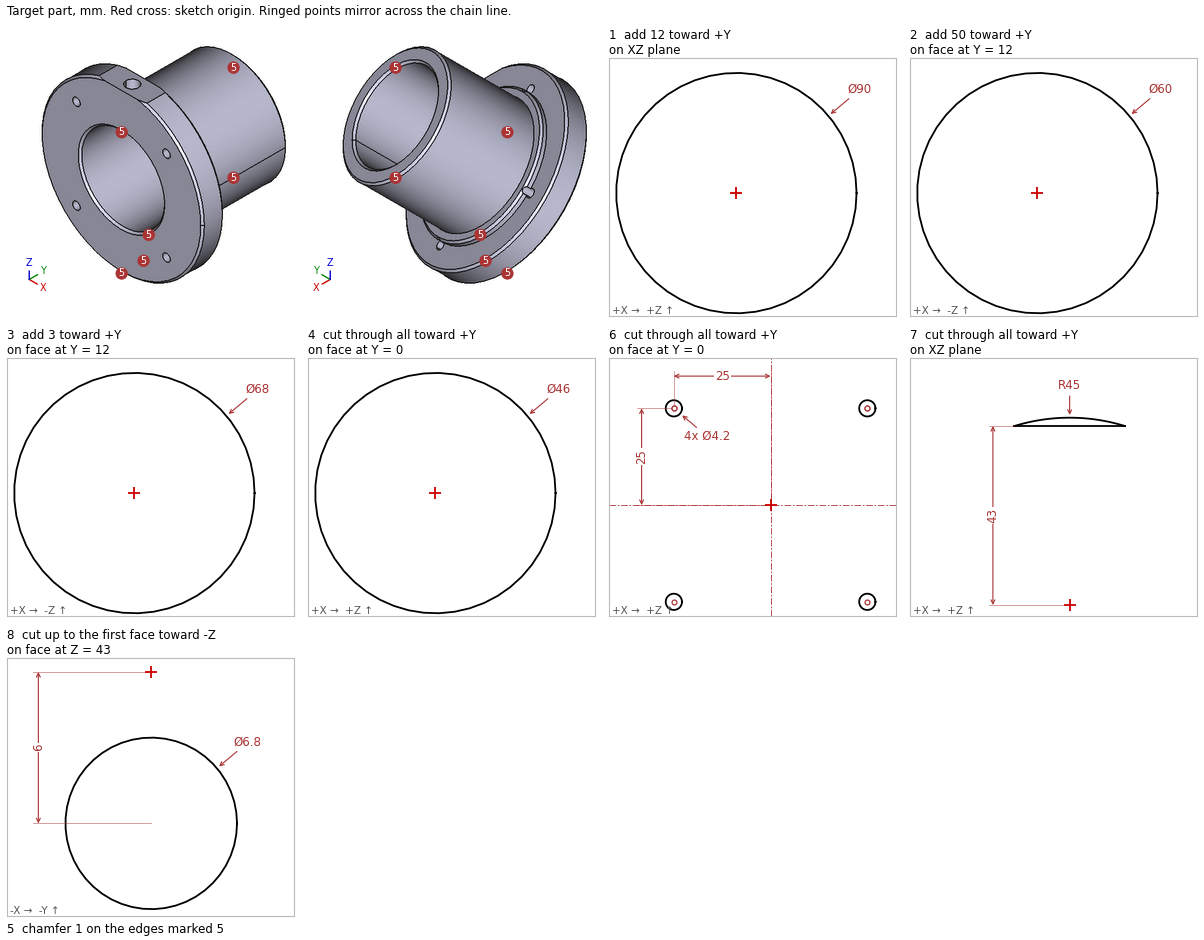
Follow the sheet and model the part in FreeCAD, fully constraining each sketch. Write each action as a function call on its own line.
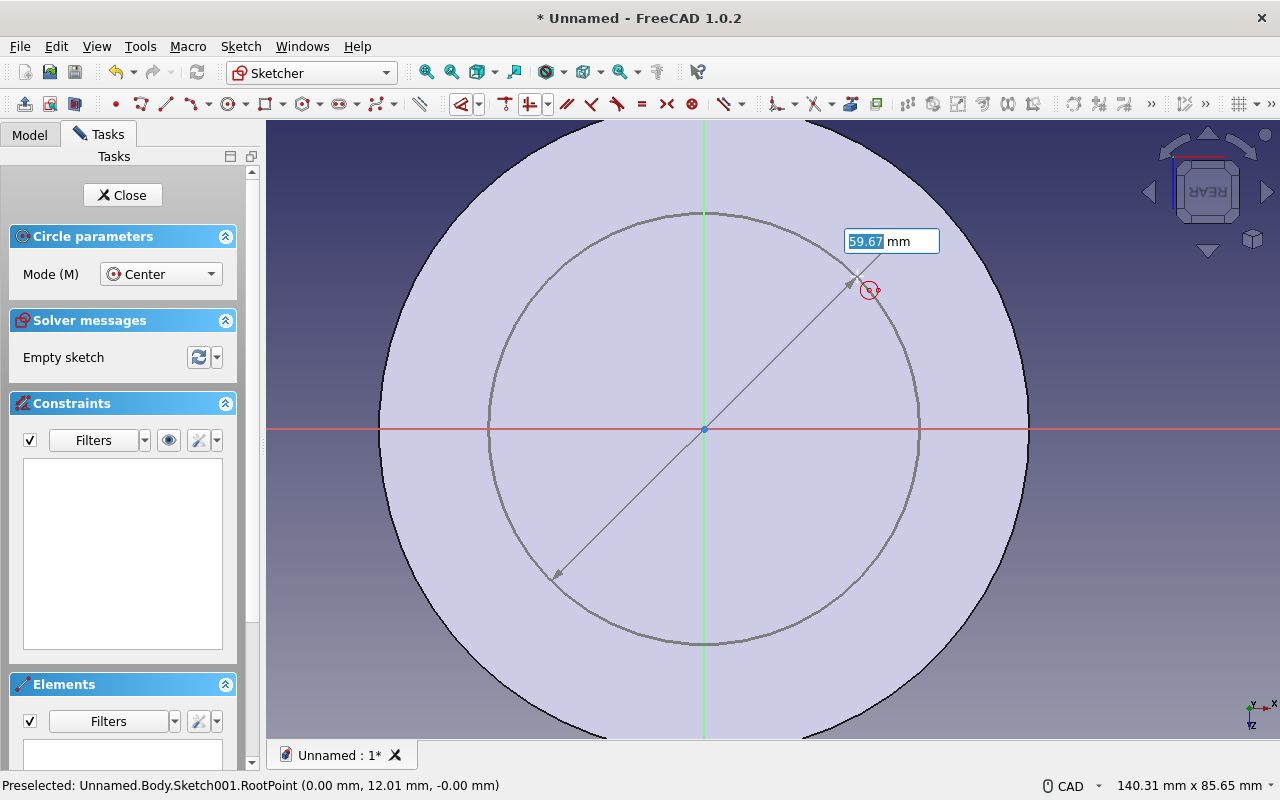
text(60)
key(Return)
key(Escape)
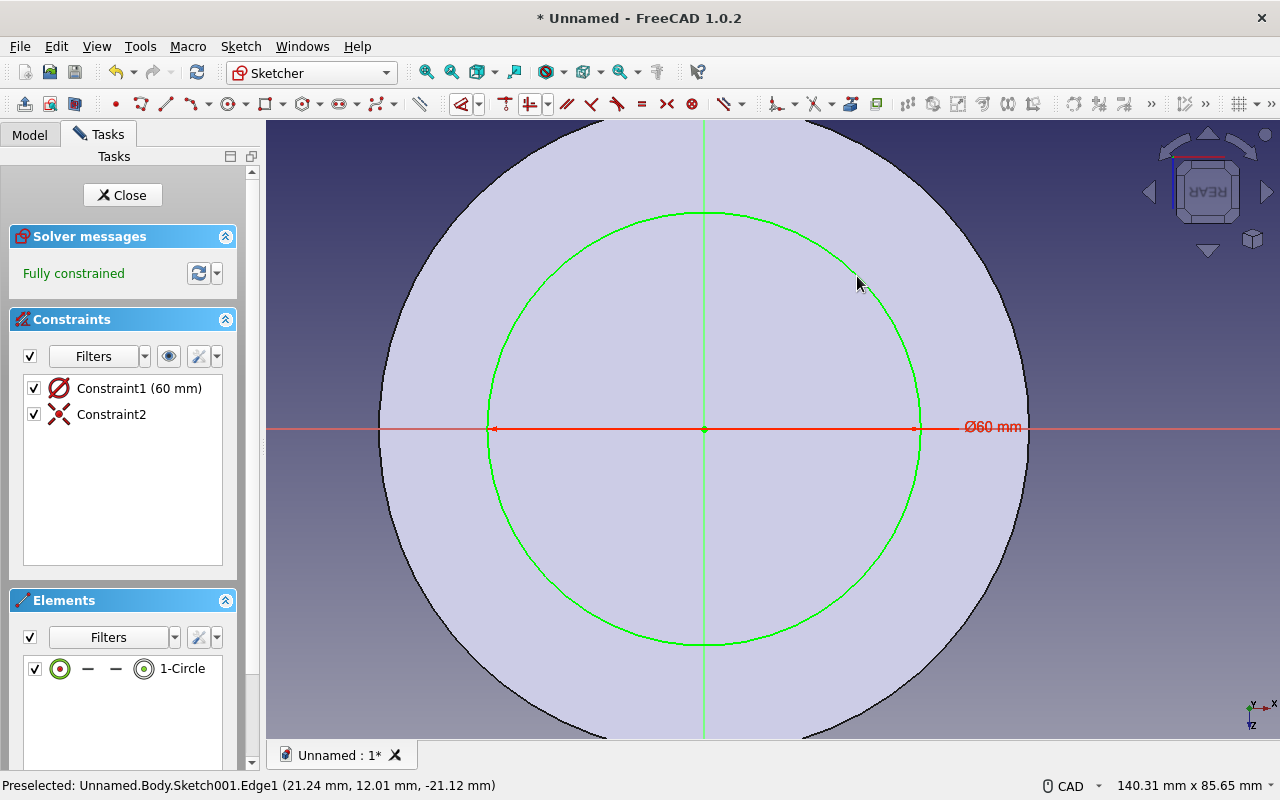
click(123, 195)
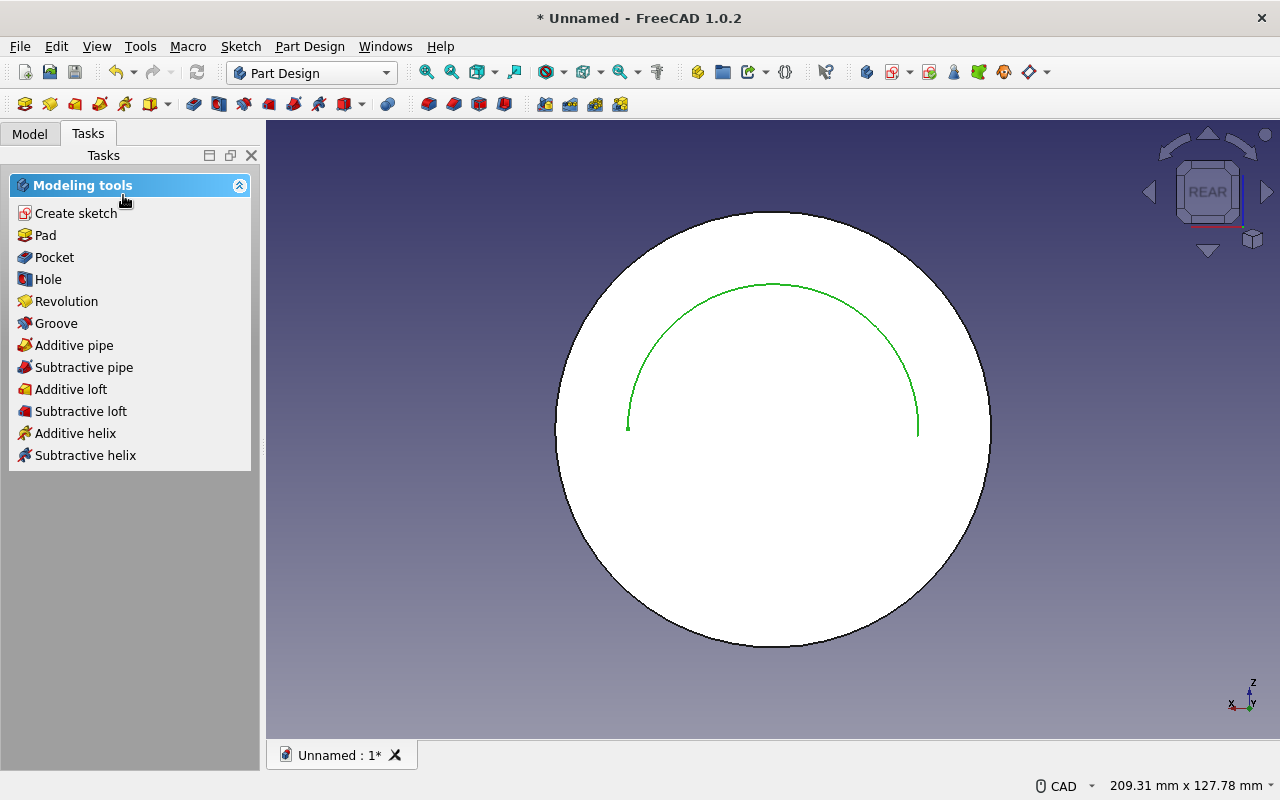
click(25, 104)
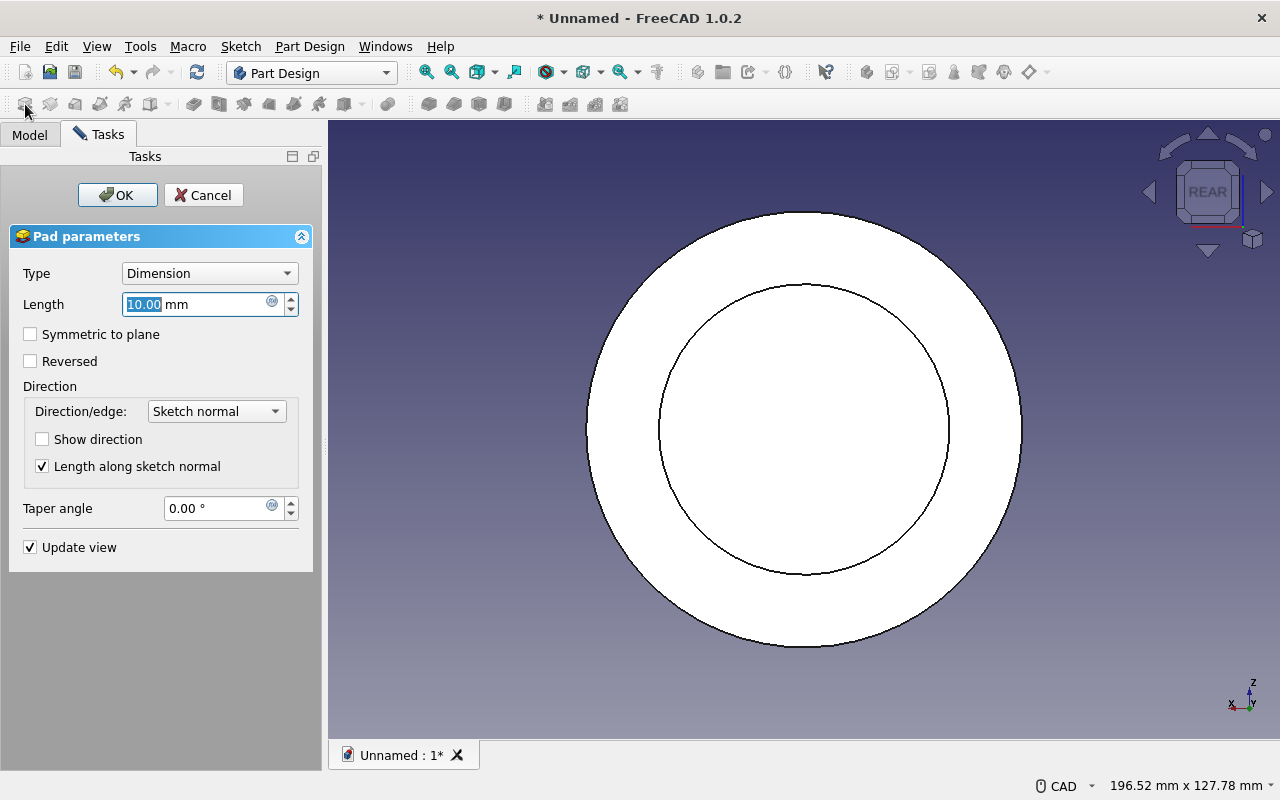
text(50)
key(Tab)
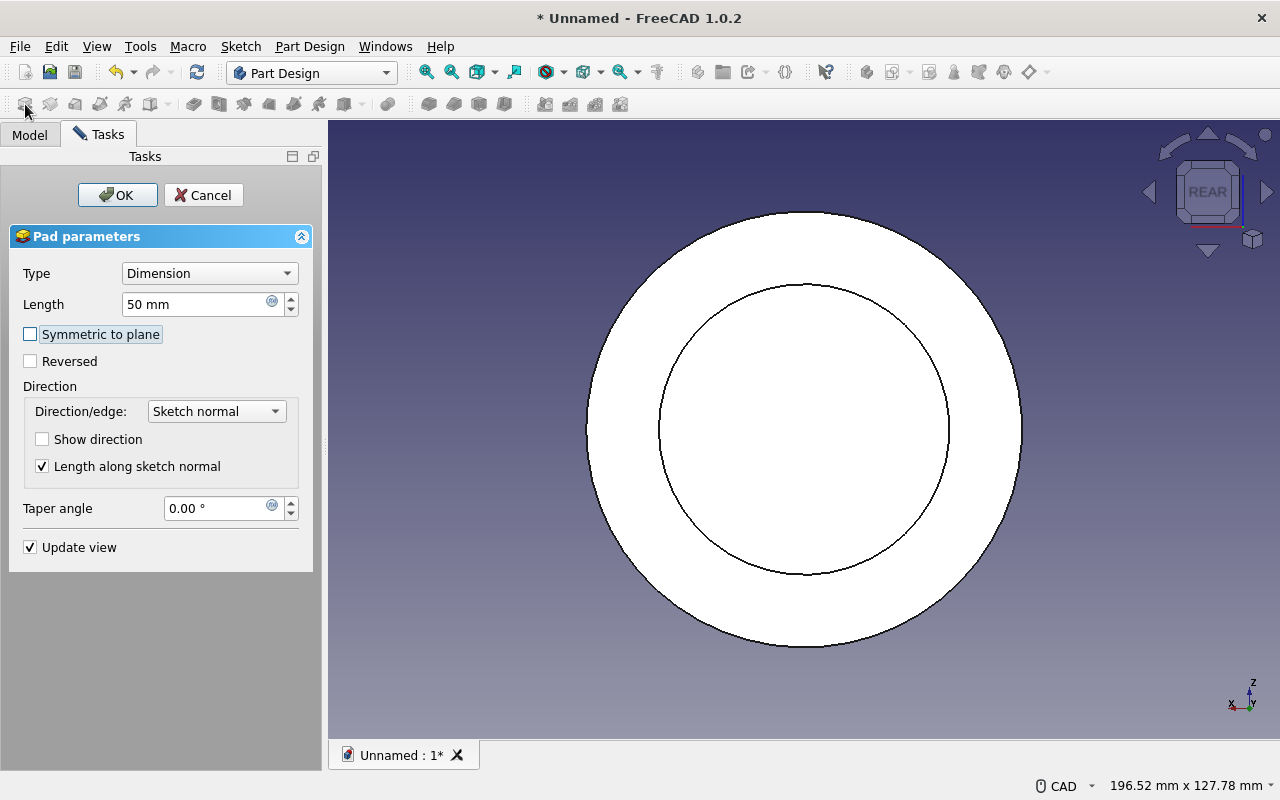
click(118, 195)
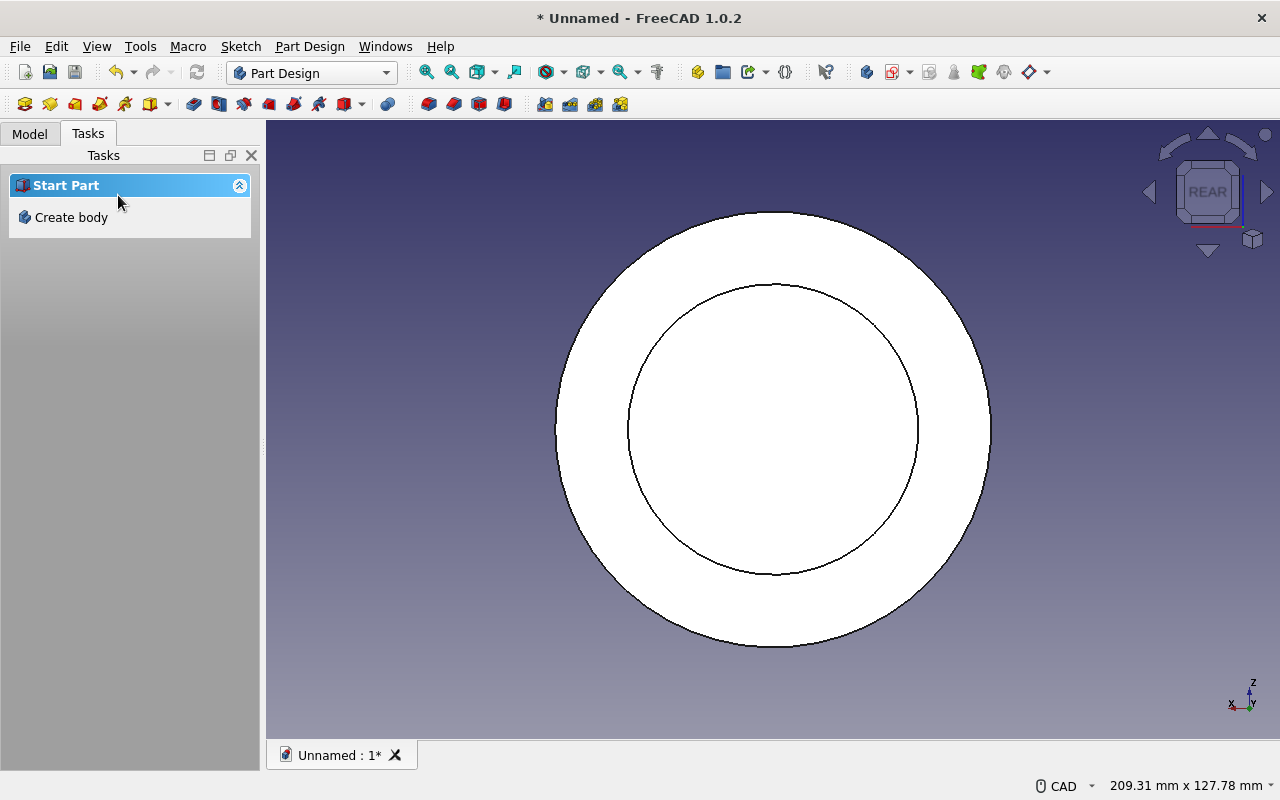
click(586, 428)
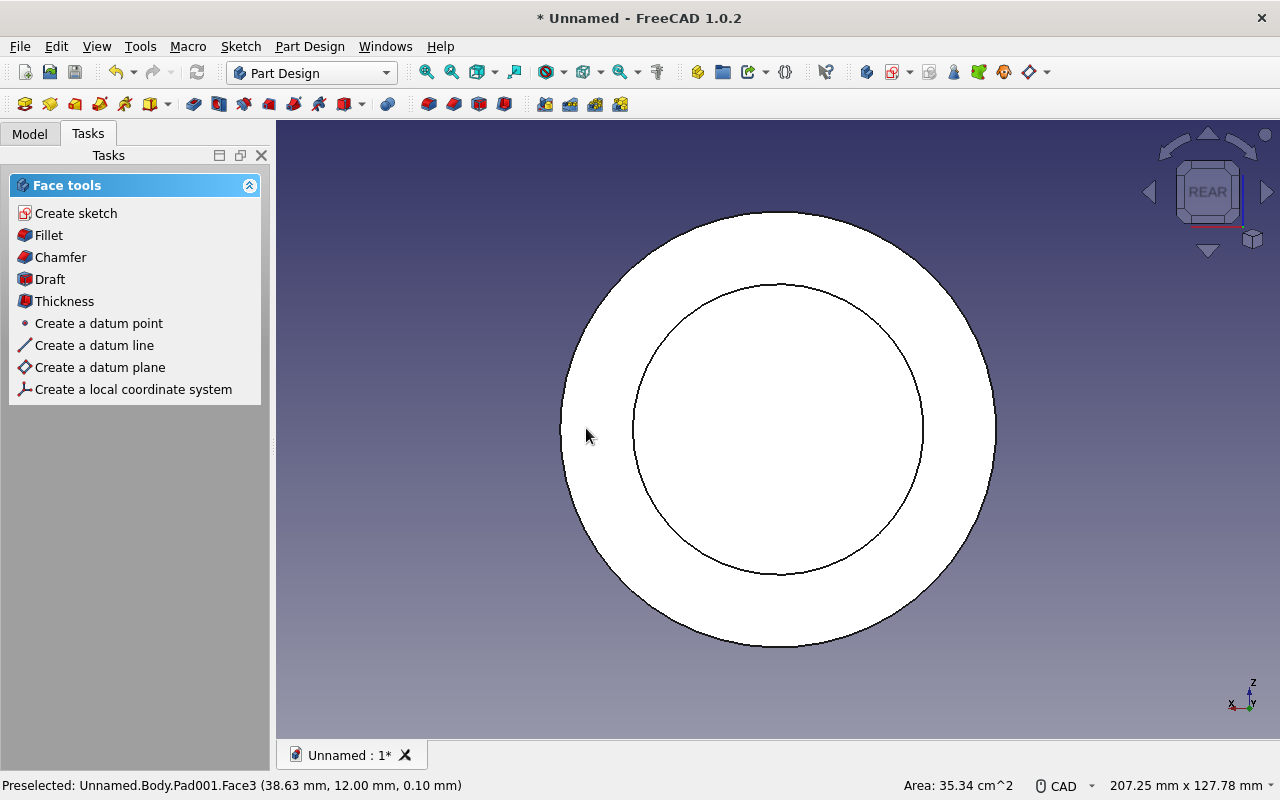
click(892, 72)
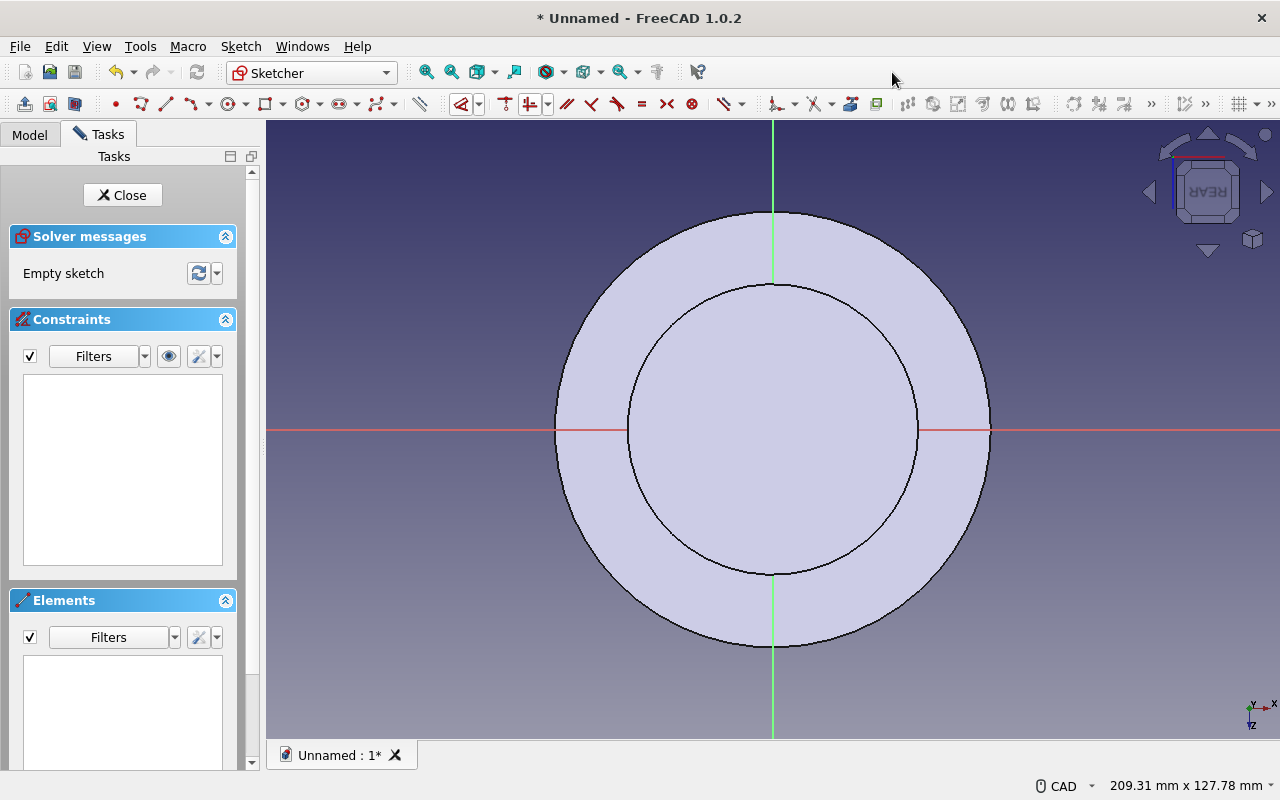
key(g)
key(c)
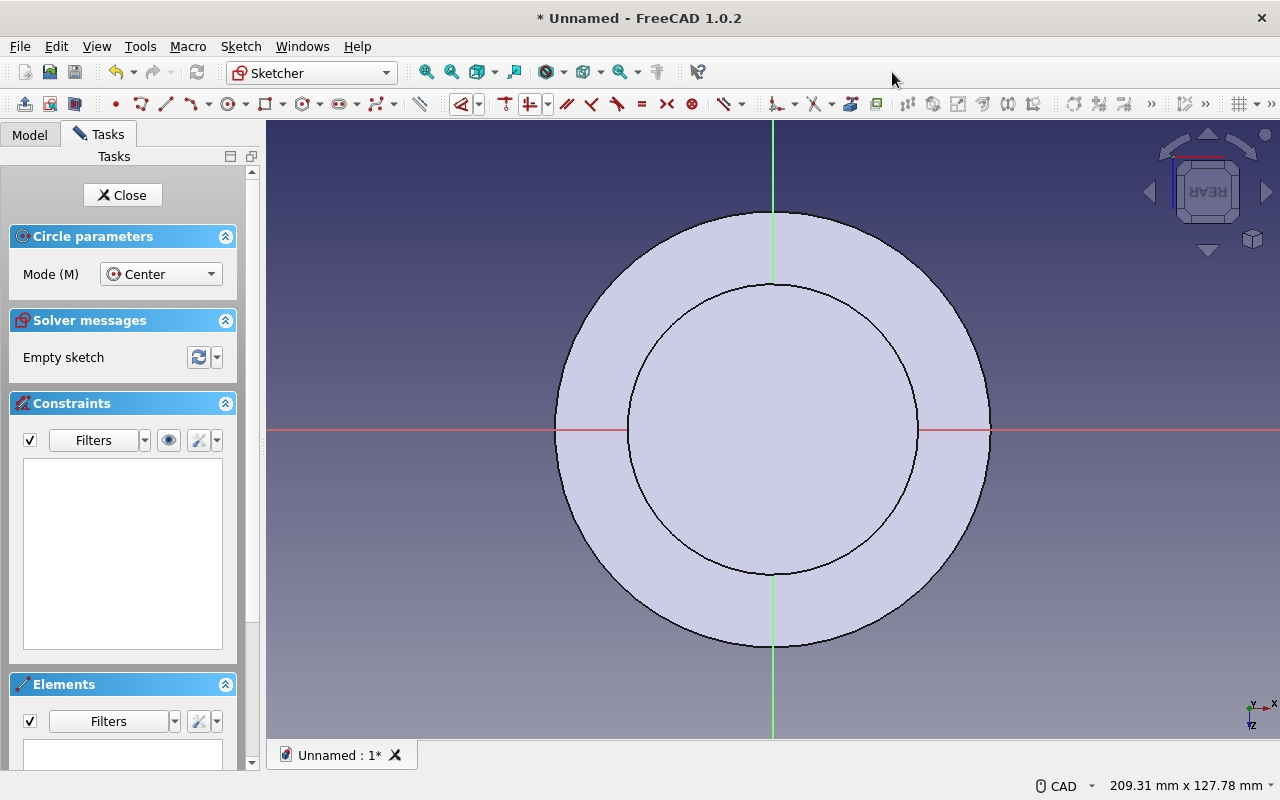
click(773, 429)
move(889, 313)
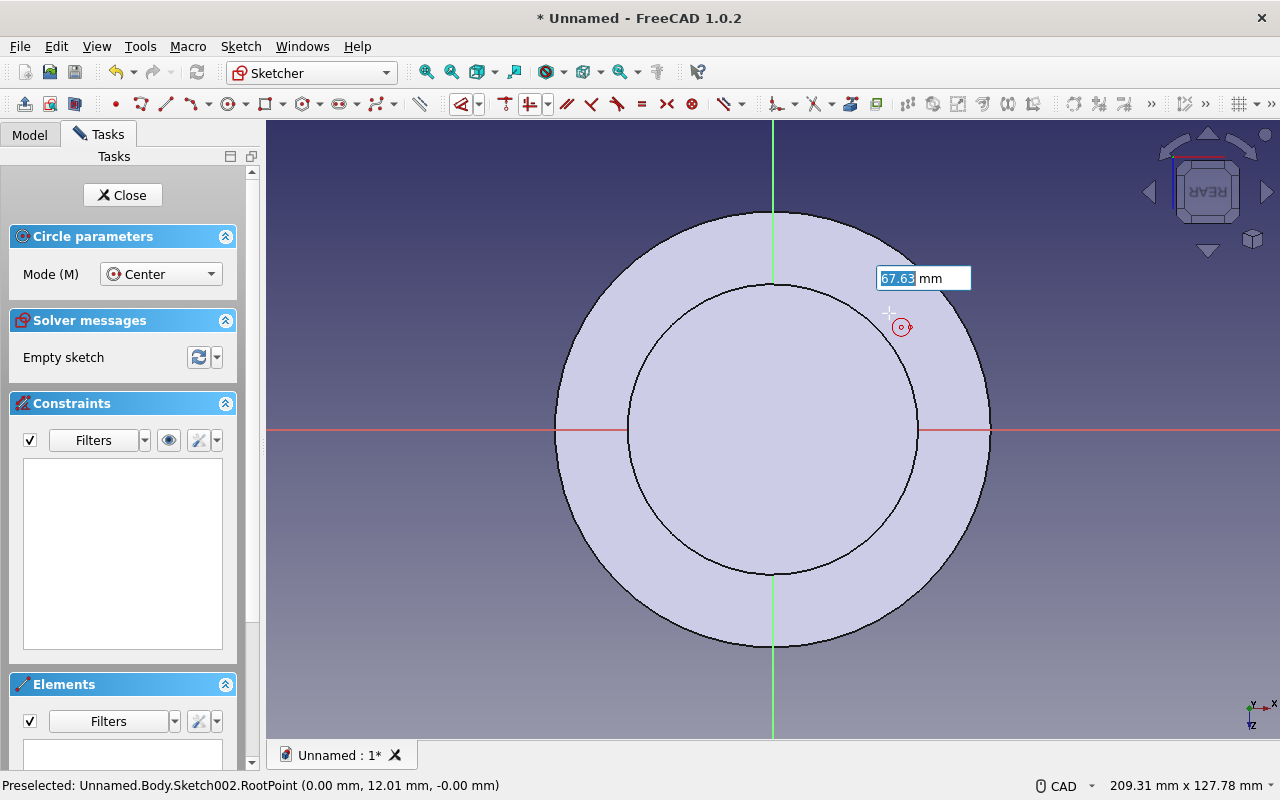
text(68)
key(Return)
key(Escape)